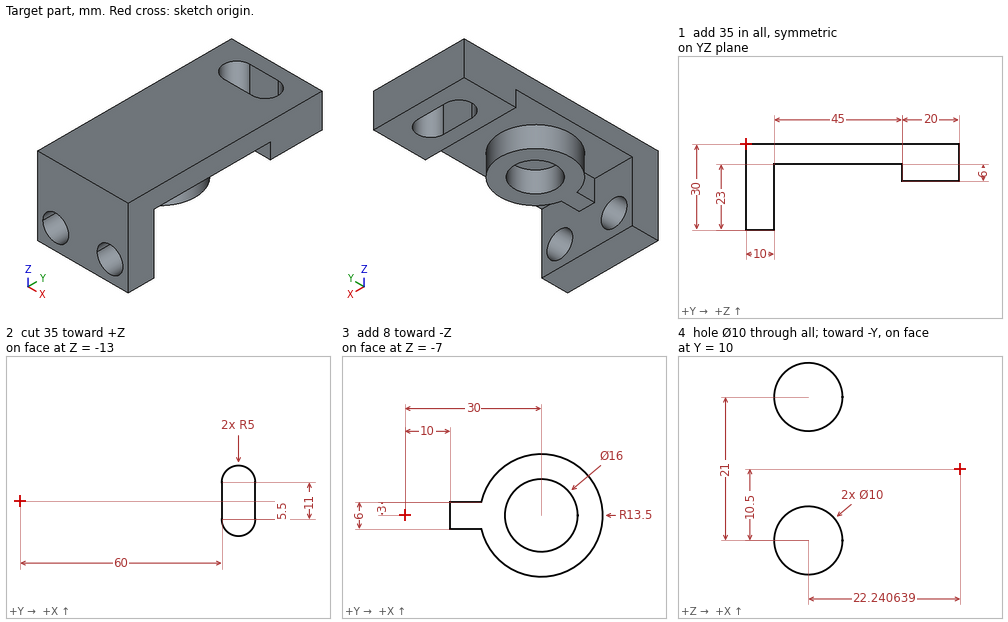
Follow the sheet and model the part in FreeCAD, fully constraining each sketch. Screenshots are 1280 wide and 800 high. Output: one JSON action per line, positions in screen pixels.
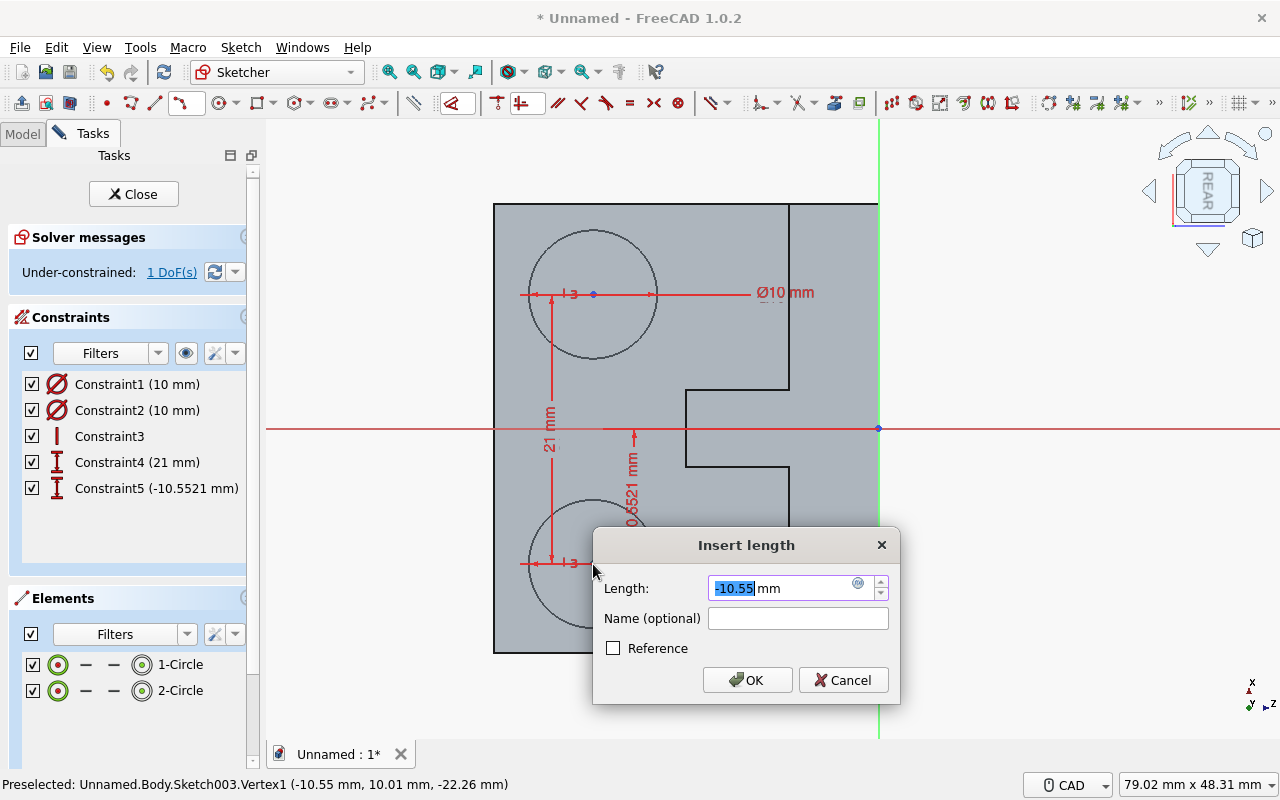
{"action": "type", "text": "-10.5"}
{"action": "key", "text": "Return"}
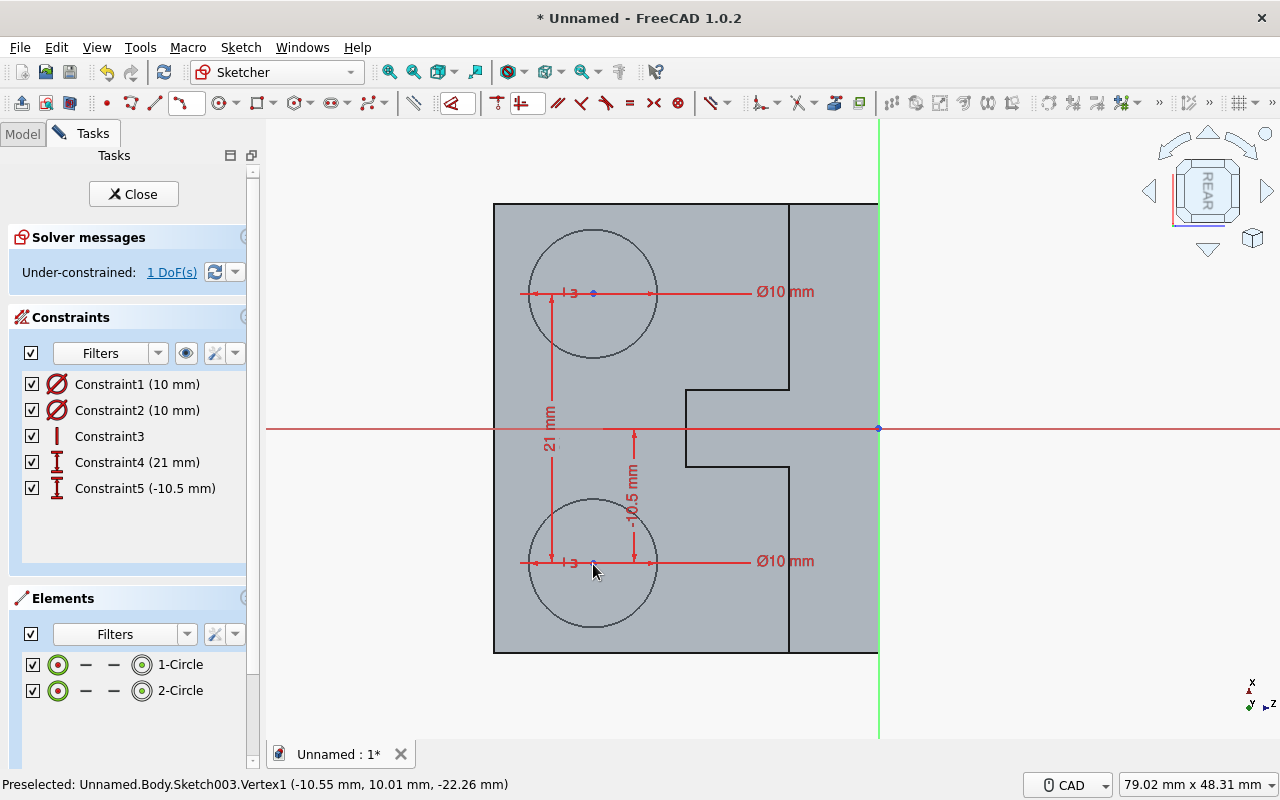
{"action": "left_click", "coordinate": [593, 563]}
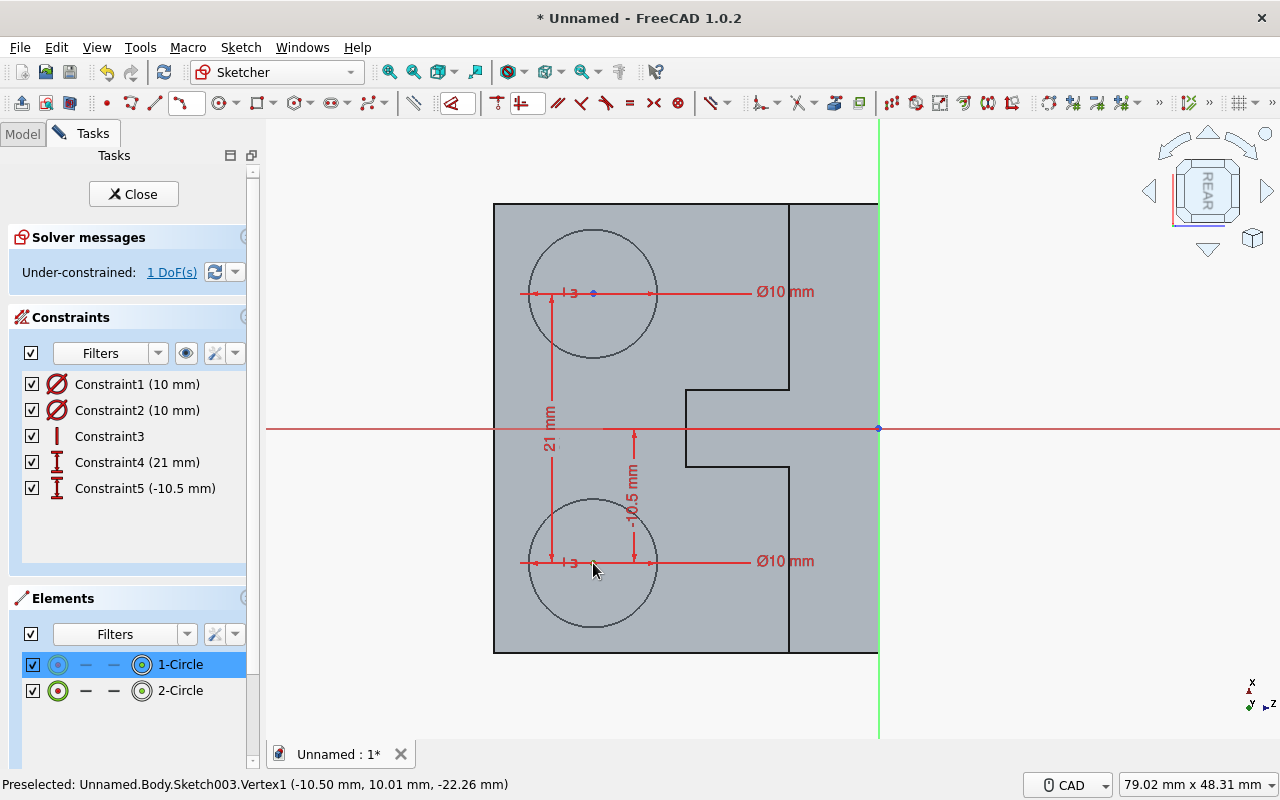
{"action": "left_click", "coordinate": [470, 104]}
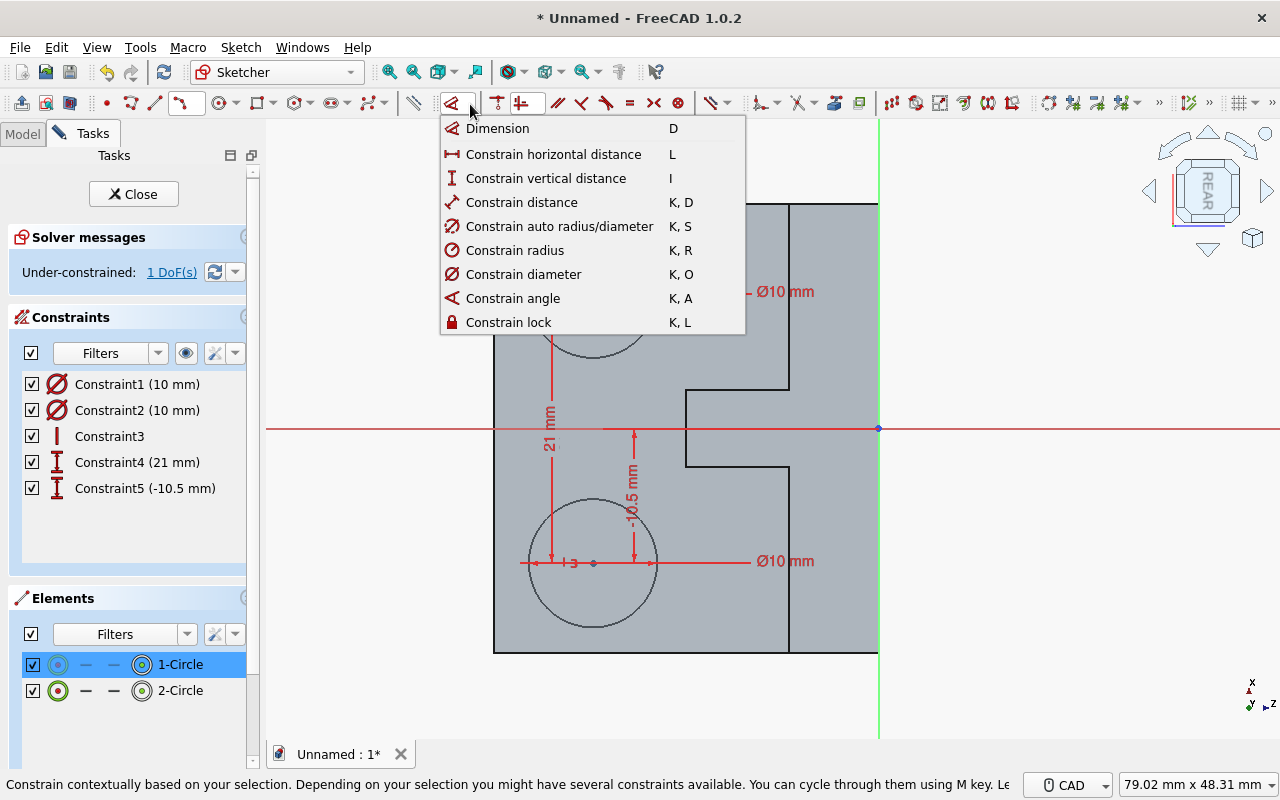
{"action": "left_click", "coordinate": [593, 154]}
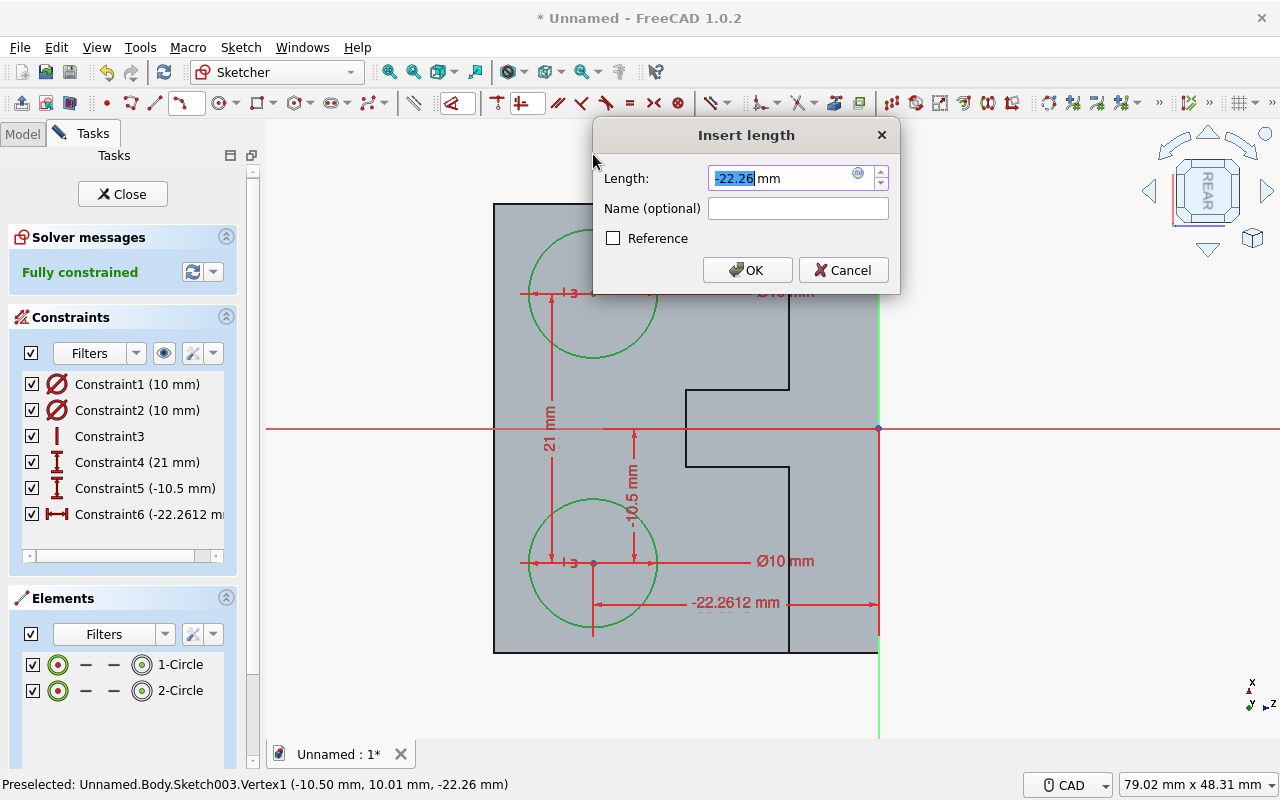
{"action": "type", "text": "-22.240639"}
{"action": "key", "text": "Return"}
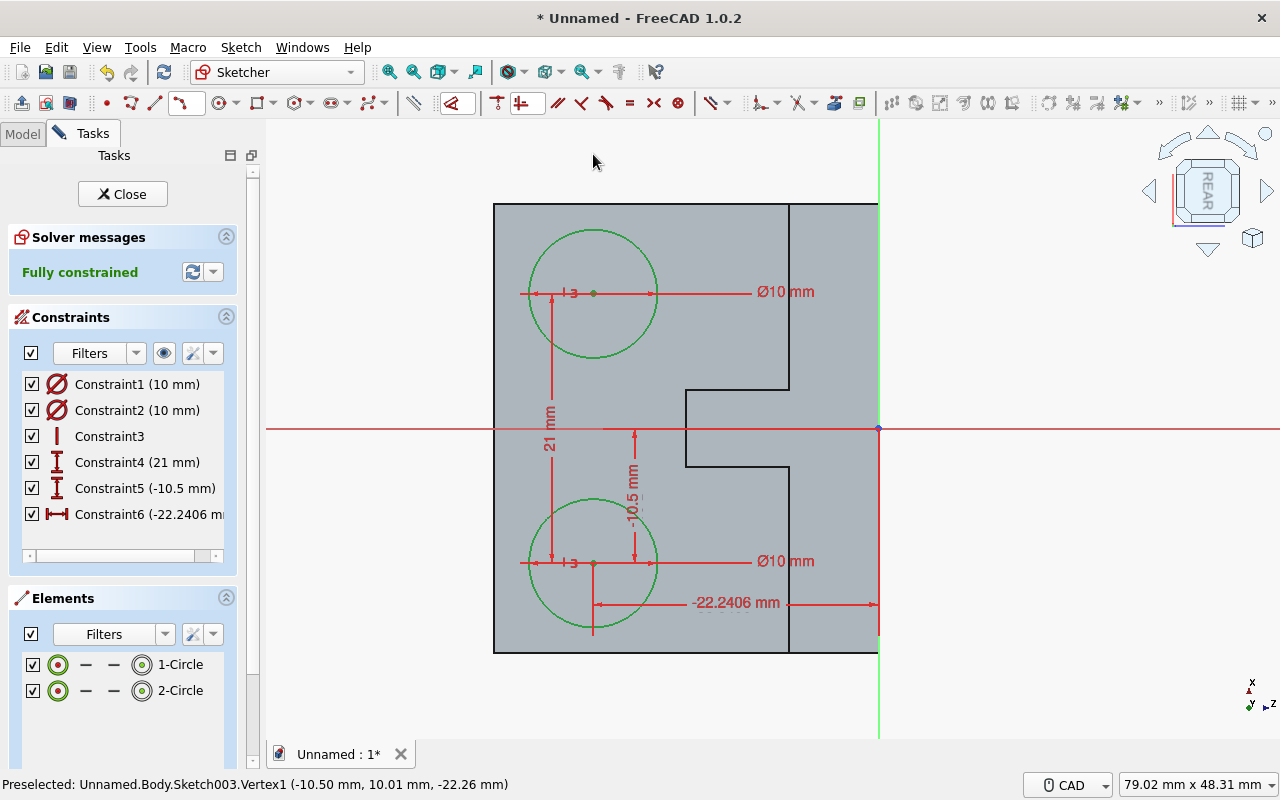
{"action": "left_click", "coordinate": [123, 194]}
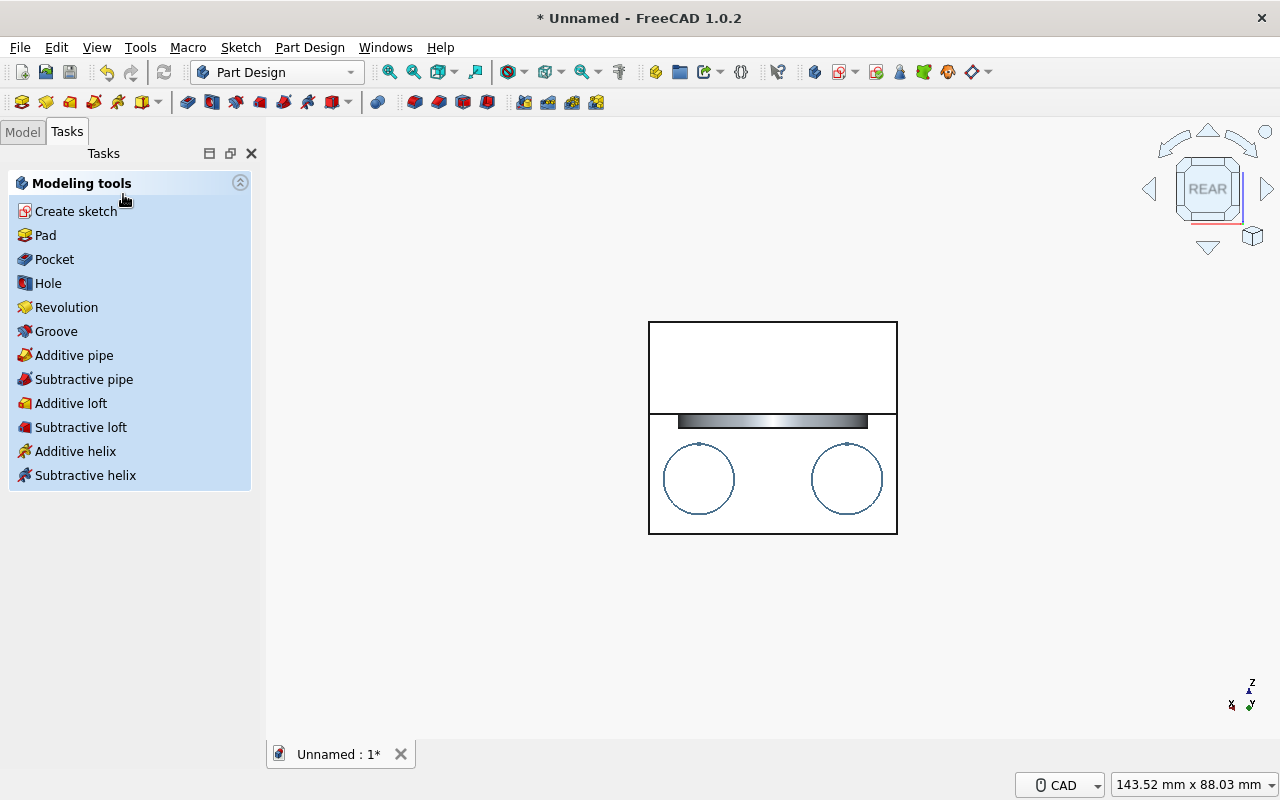
{"action": "left_click", "coordinate": [212, 102]}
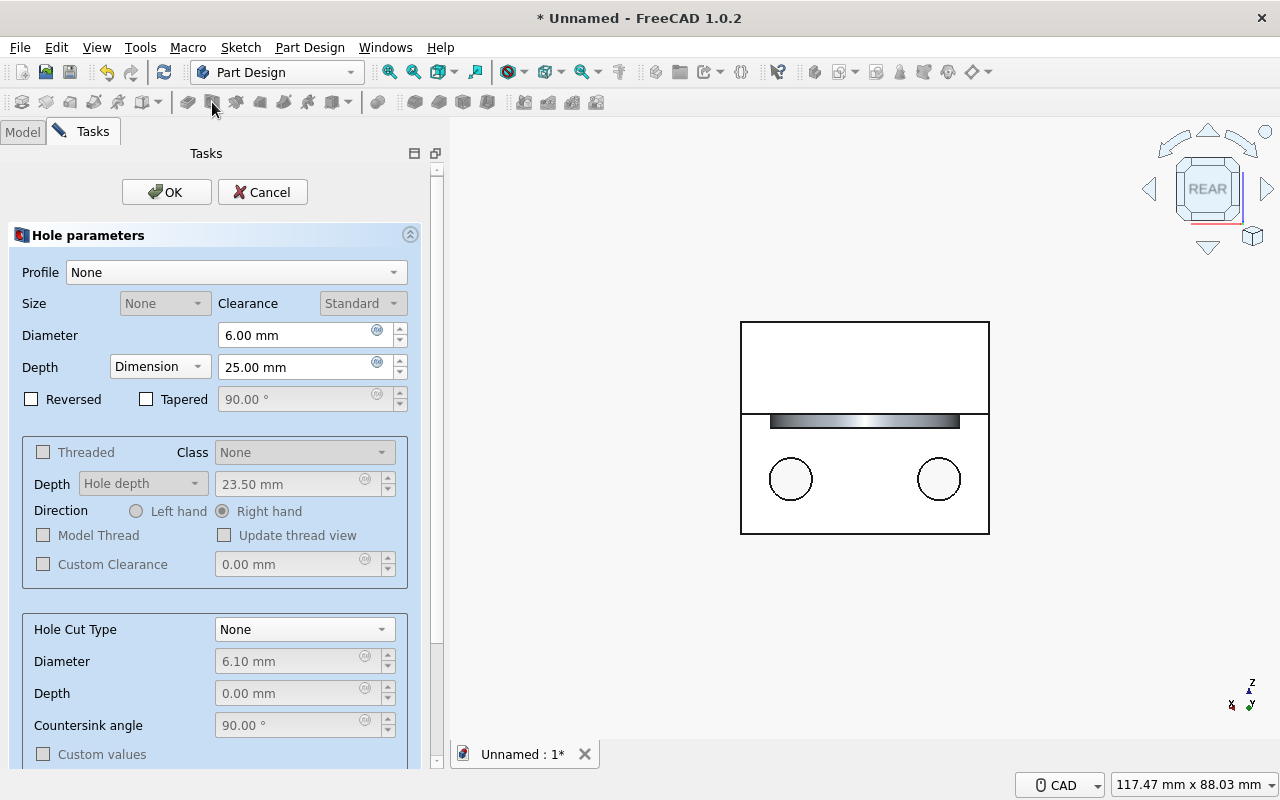
{"action": "triple_click", "coordinate": [305, 335]}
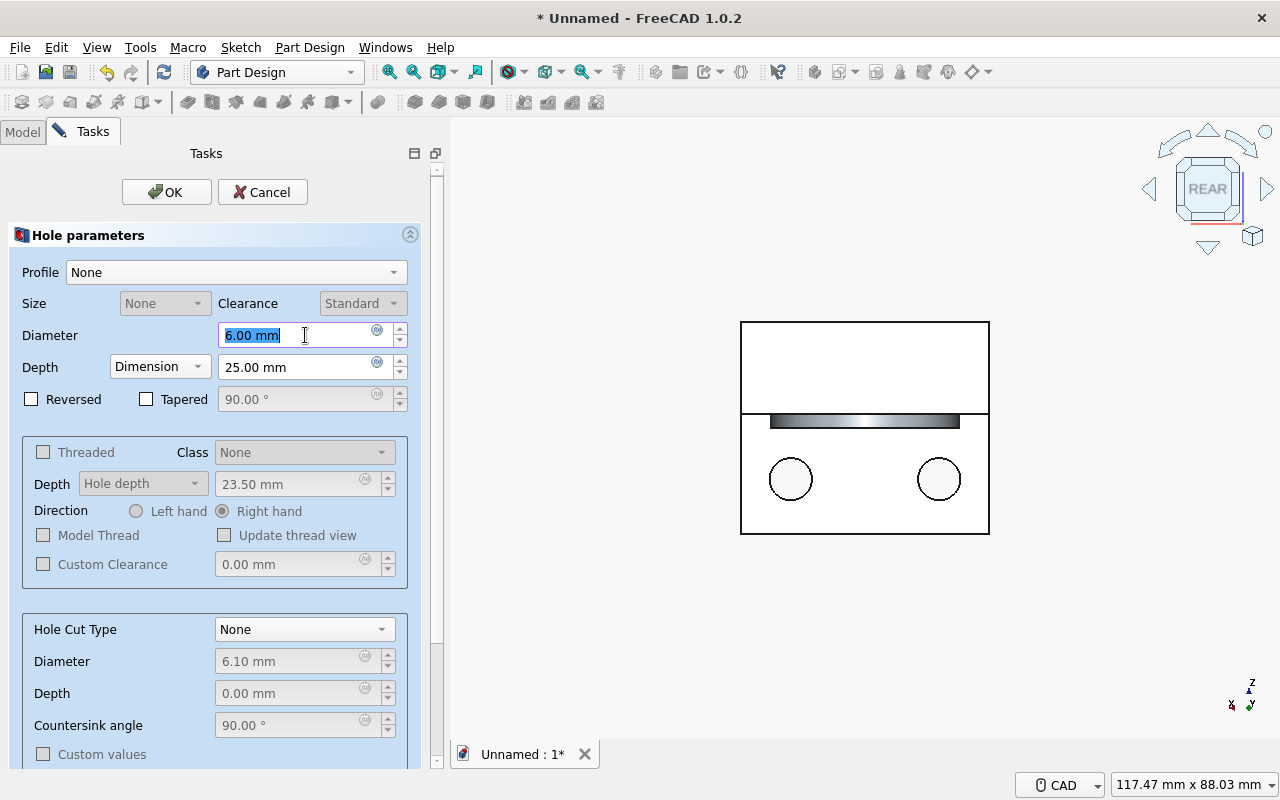
{"action": "type", "text": "10"}
{"action": "key", "text": "Tab"}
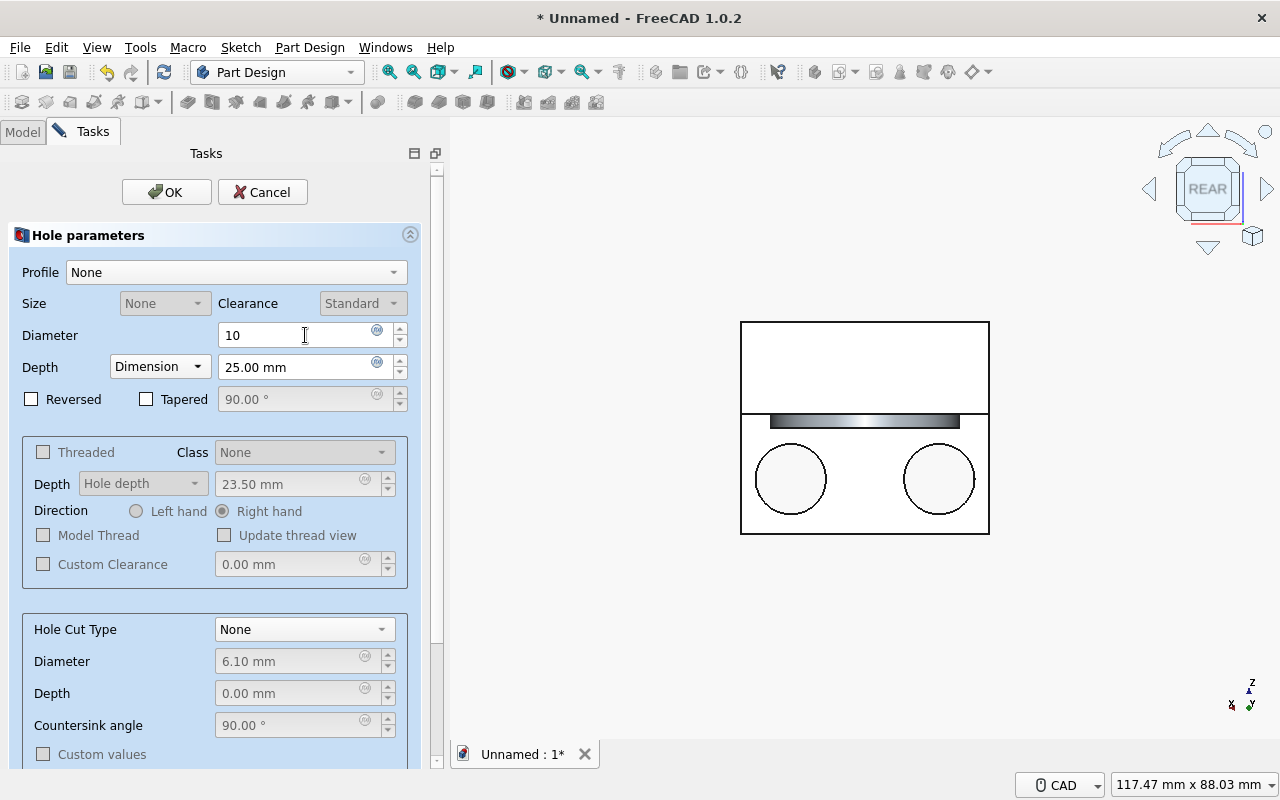
{"action": "left_click", "coordinate": [161, 366]}